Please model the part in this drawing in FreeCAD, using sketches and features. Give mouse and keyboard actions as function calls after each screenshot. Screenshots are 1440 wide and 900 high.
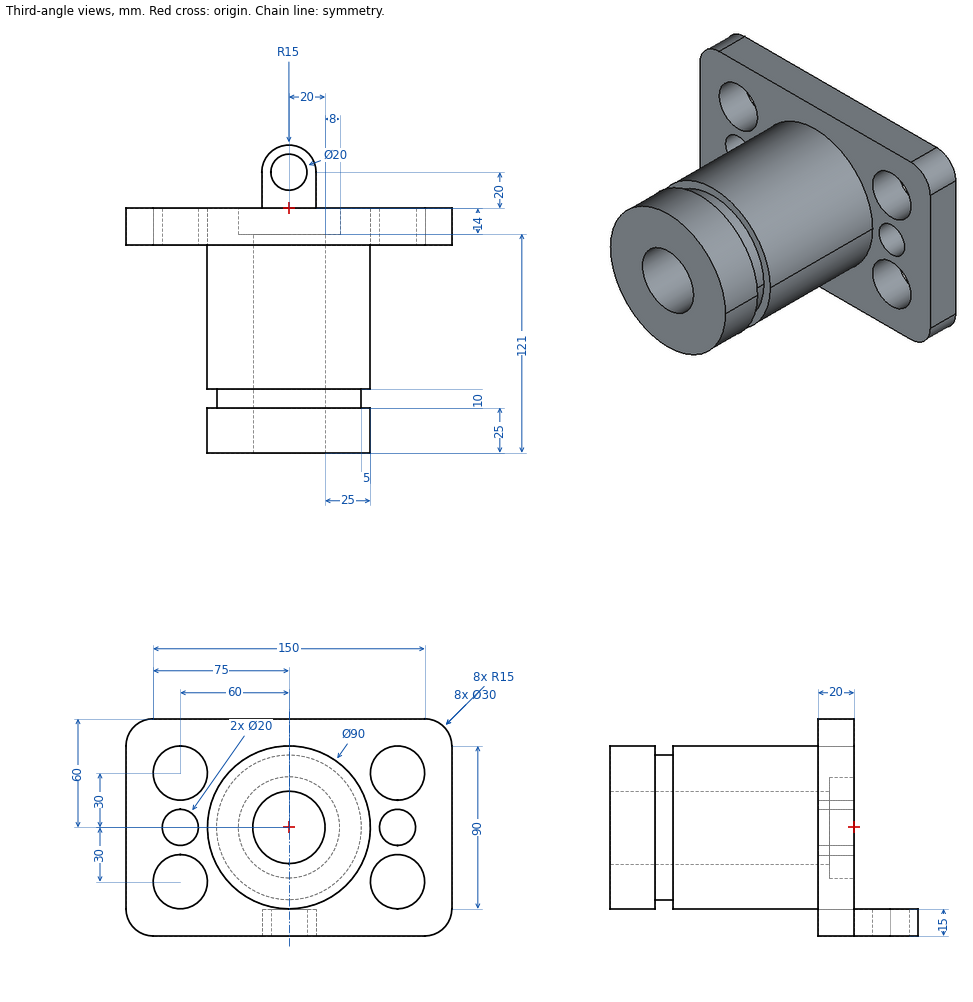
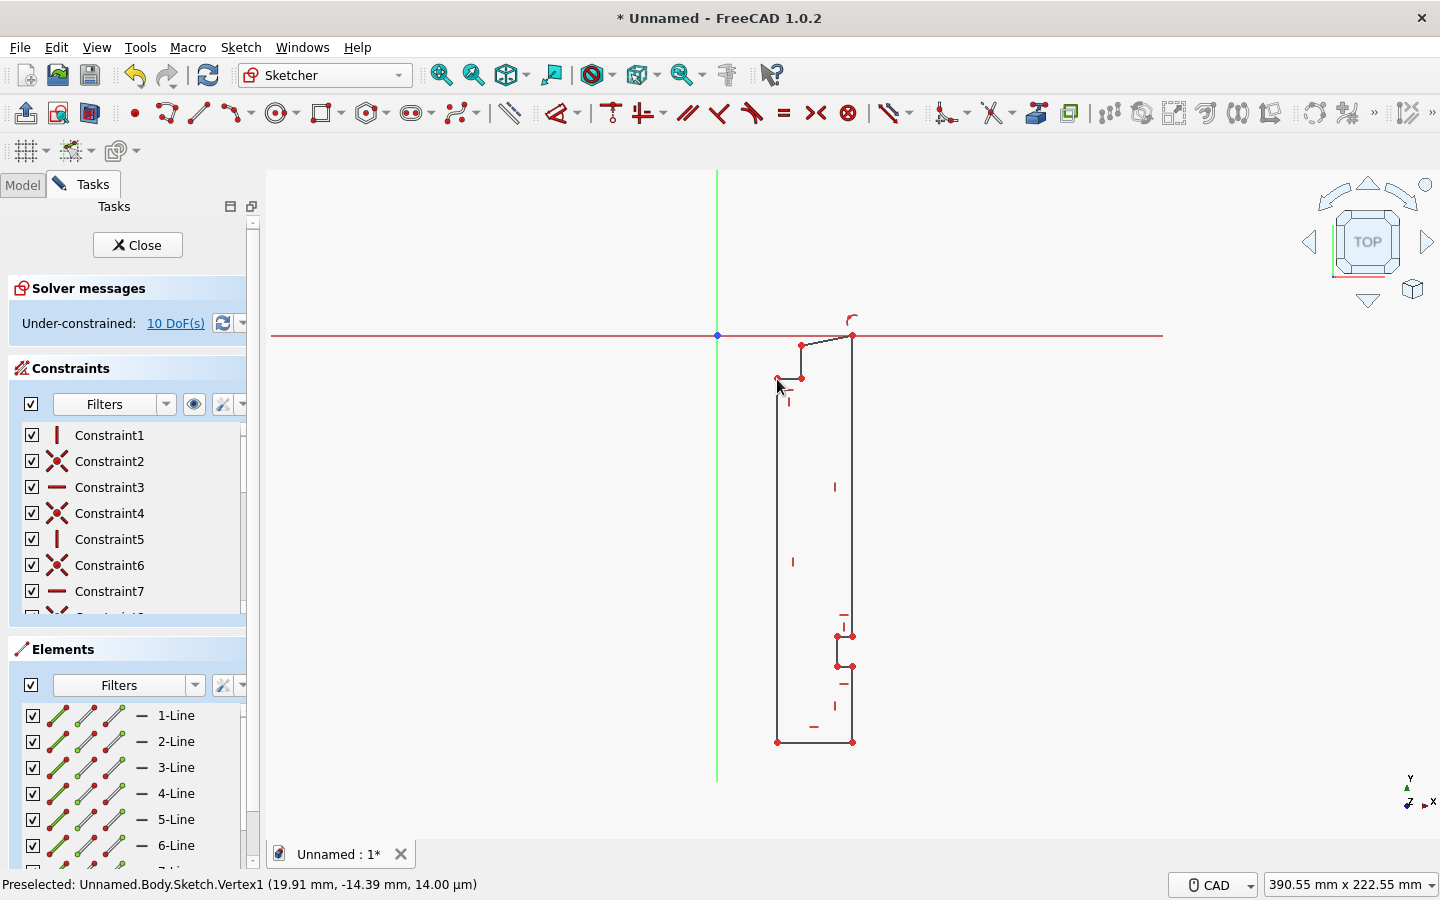
click(837, 339)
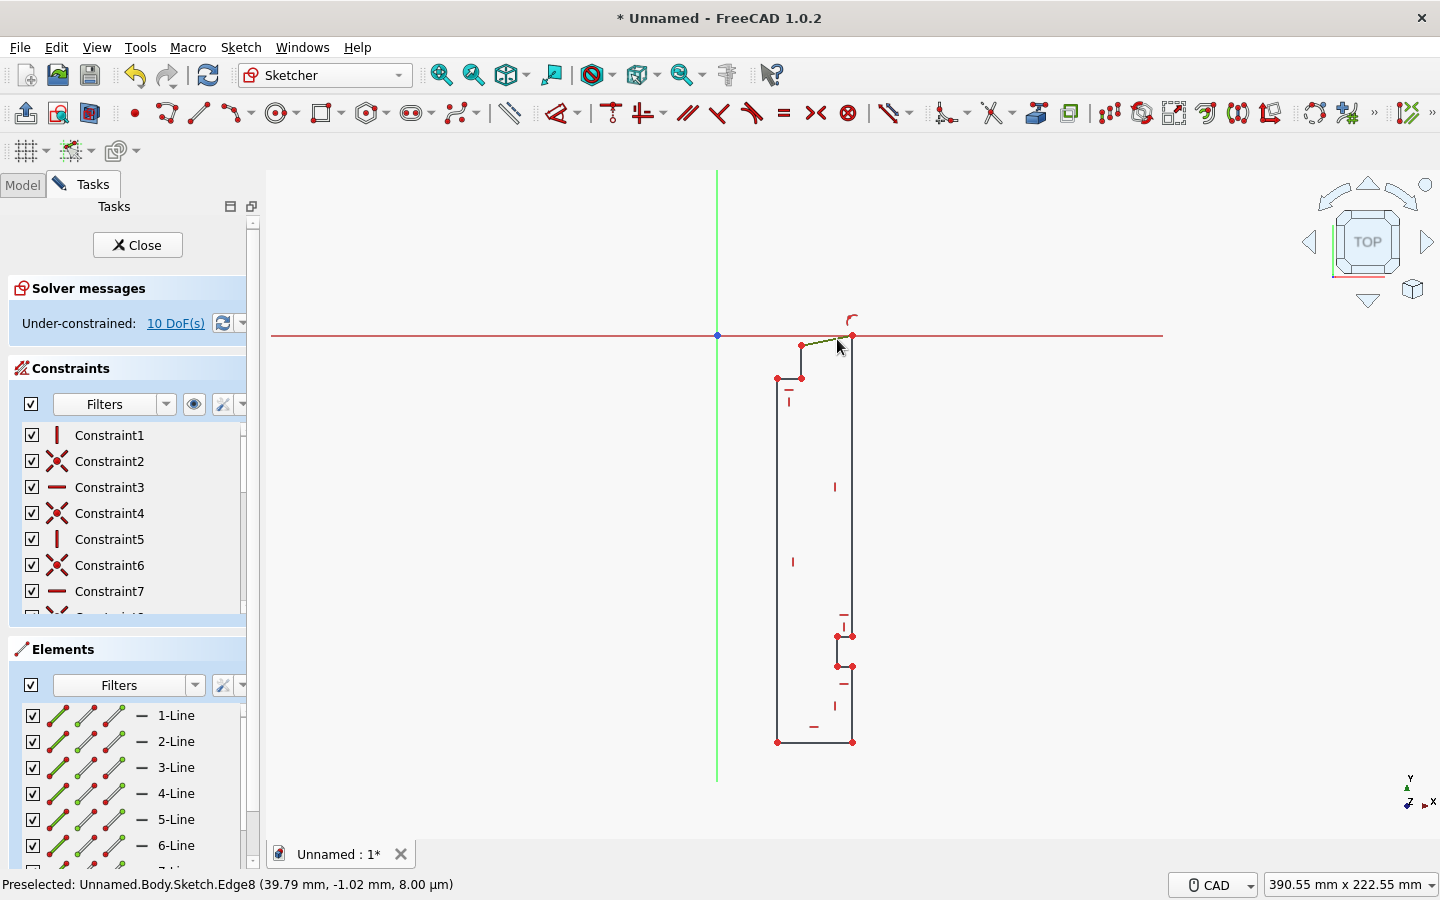
key(h)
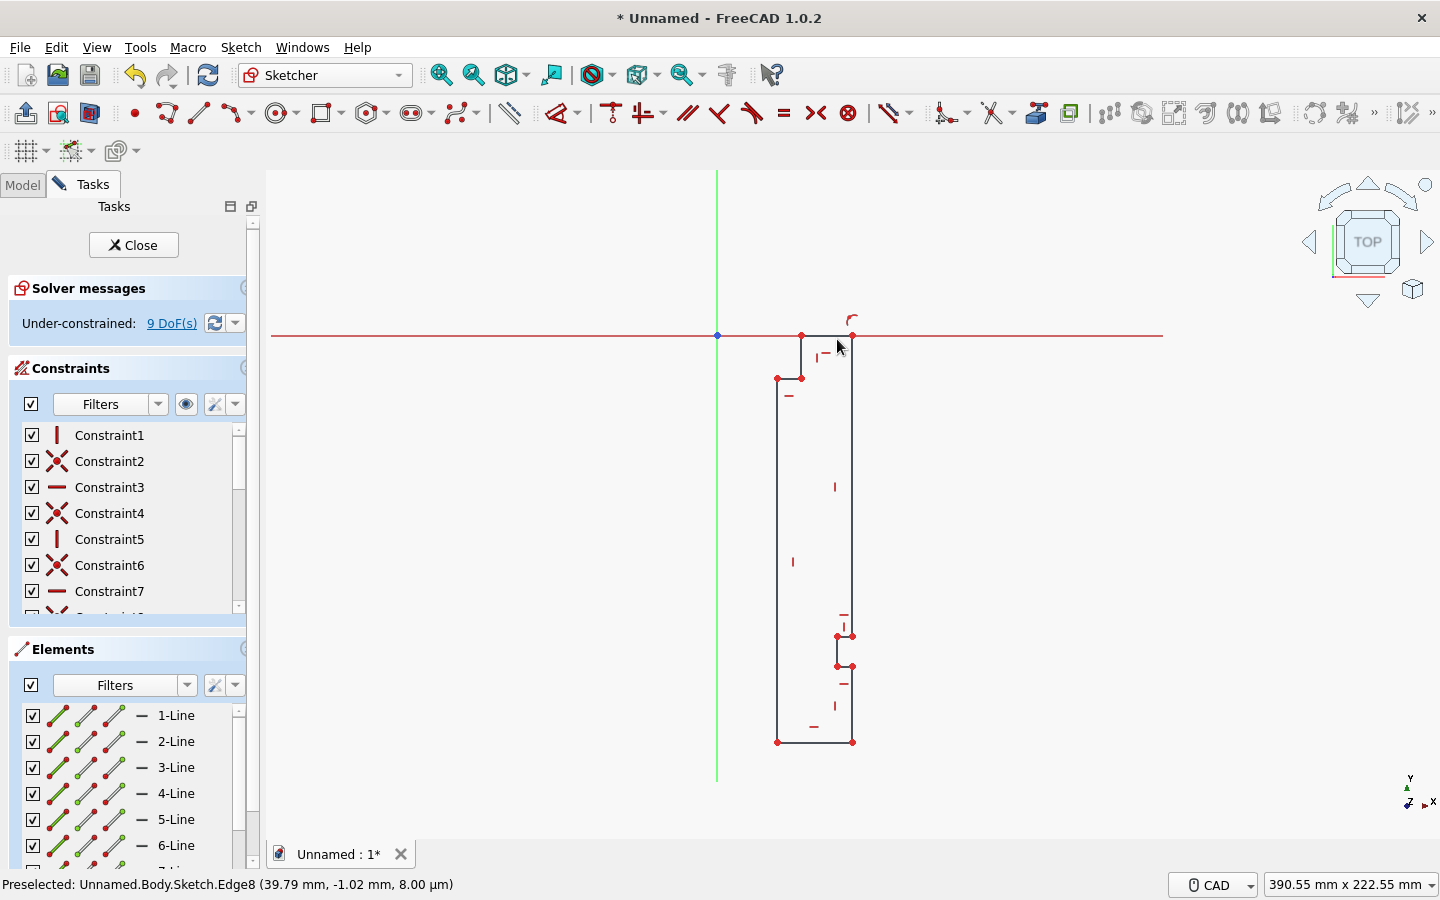
click(556, 114)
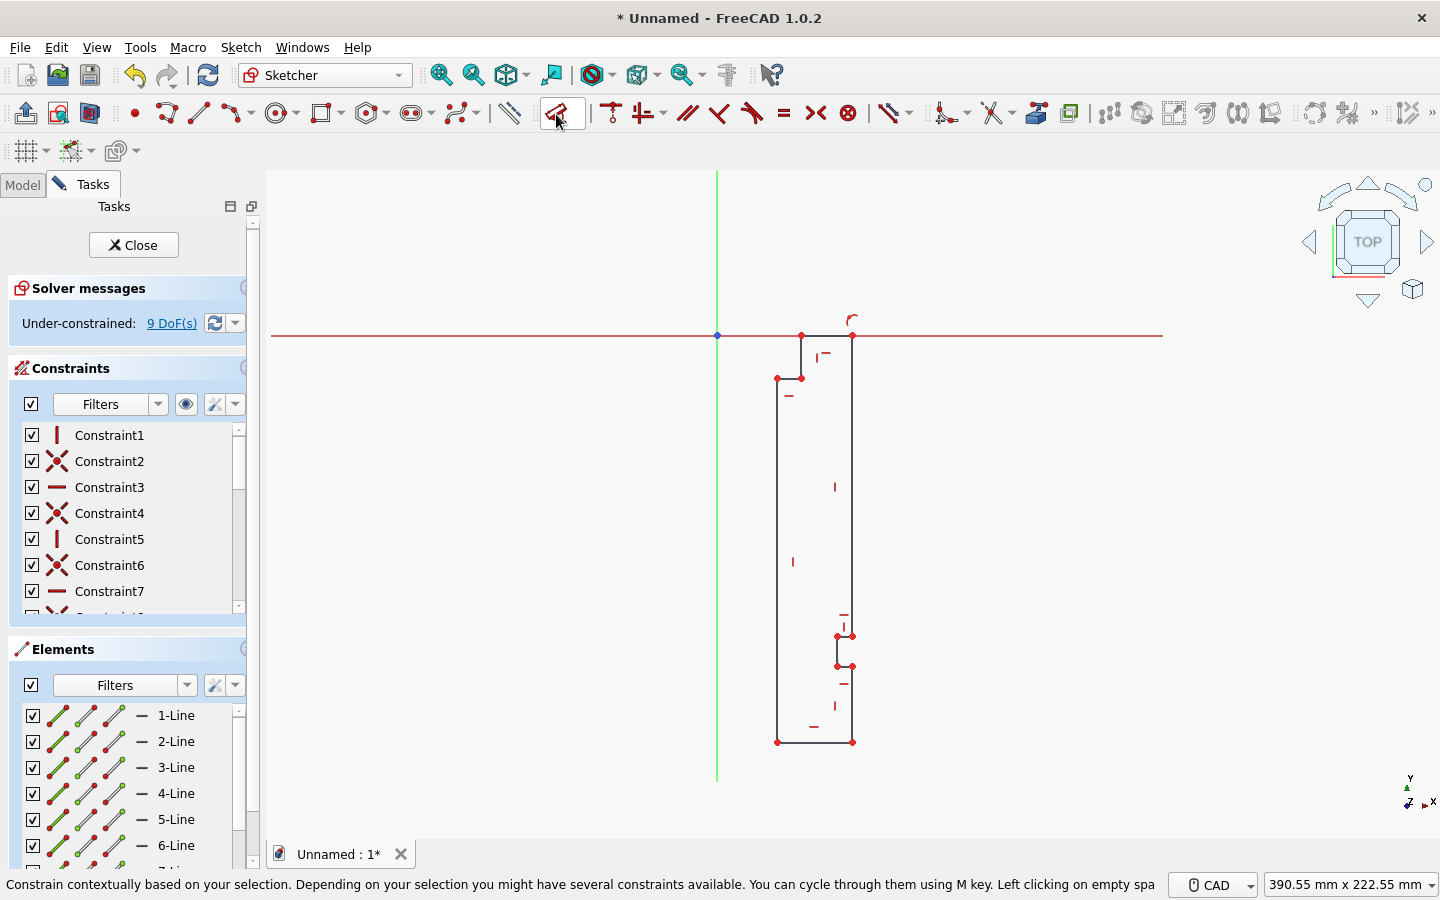
scroll(845, 667, up, 5)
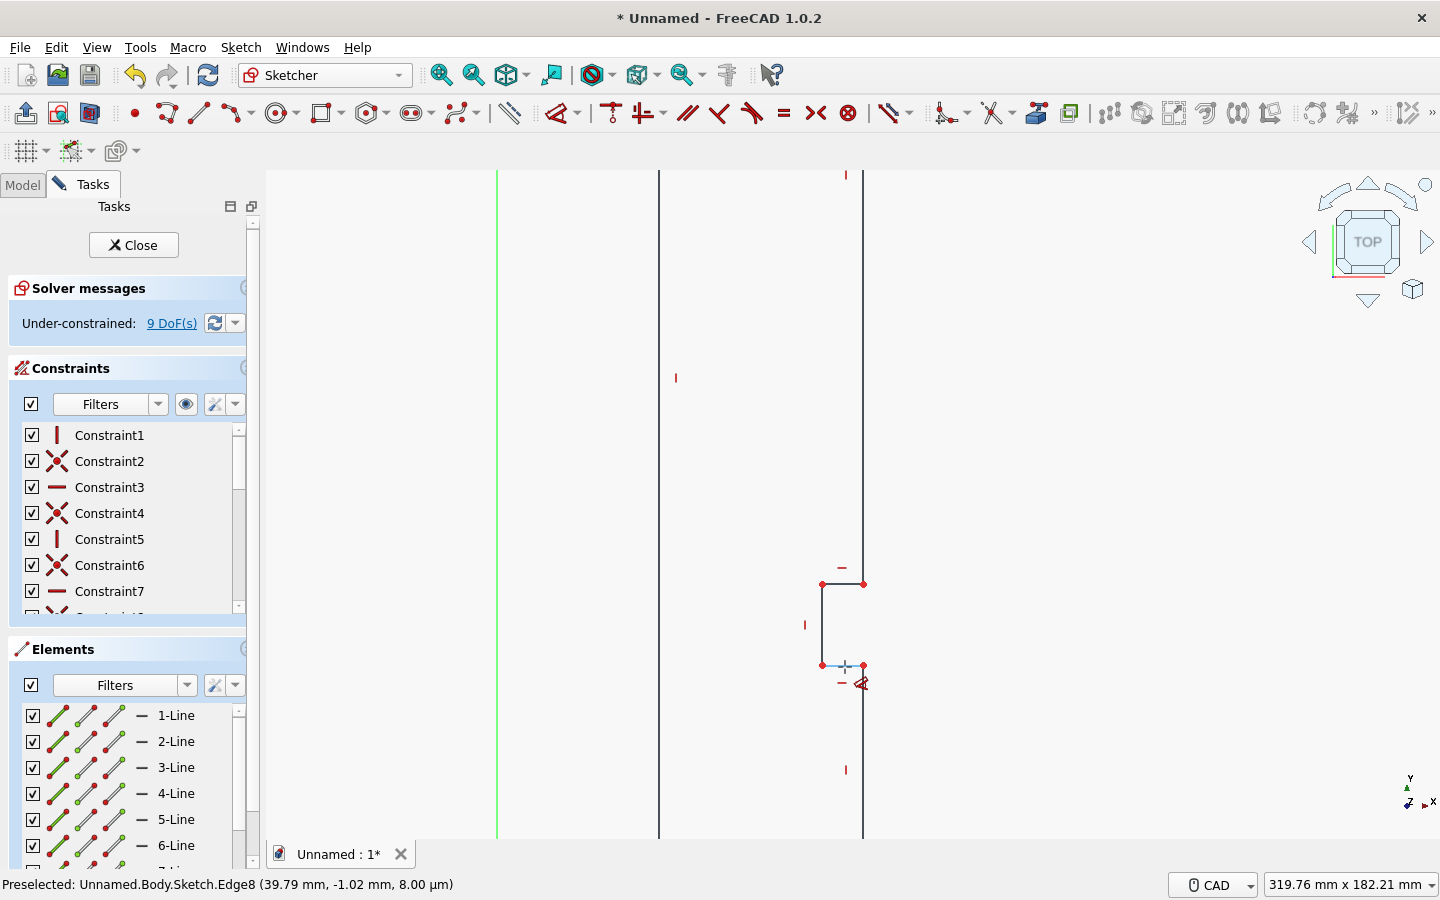
click(843, 666)
click(843, 700)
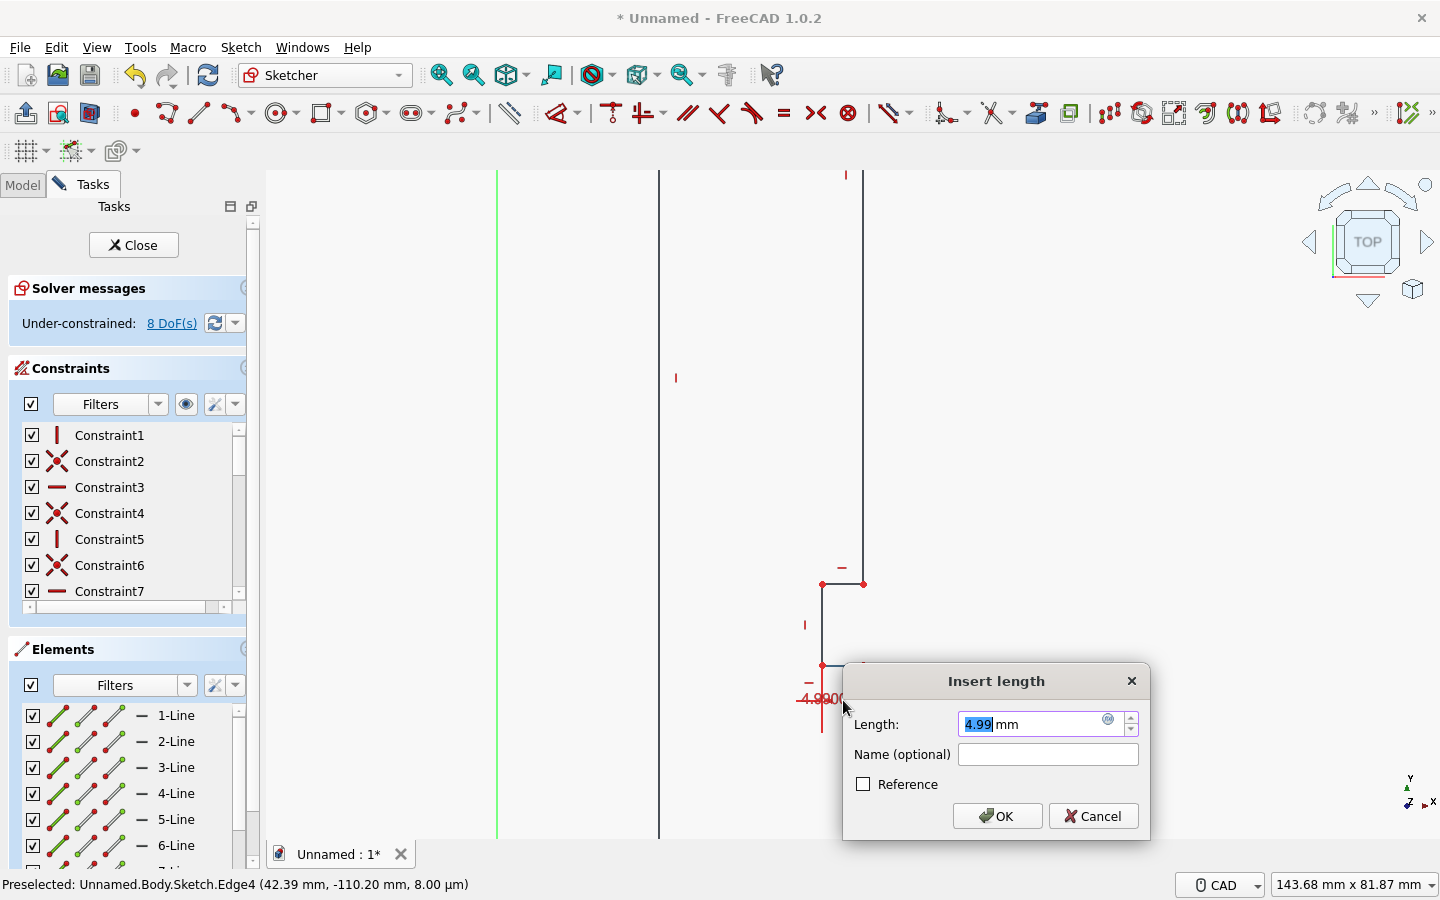
text(5)
key(Return)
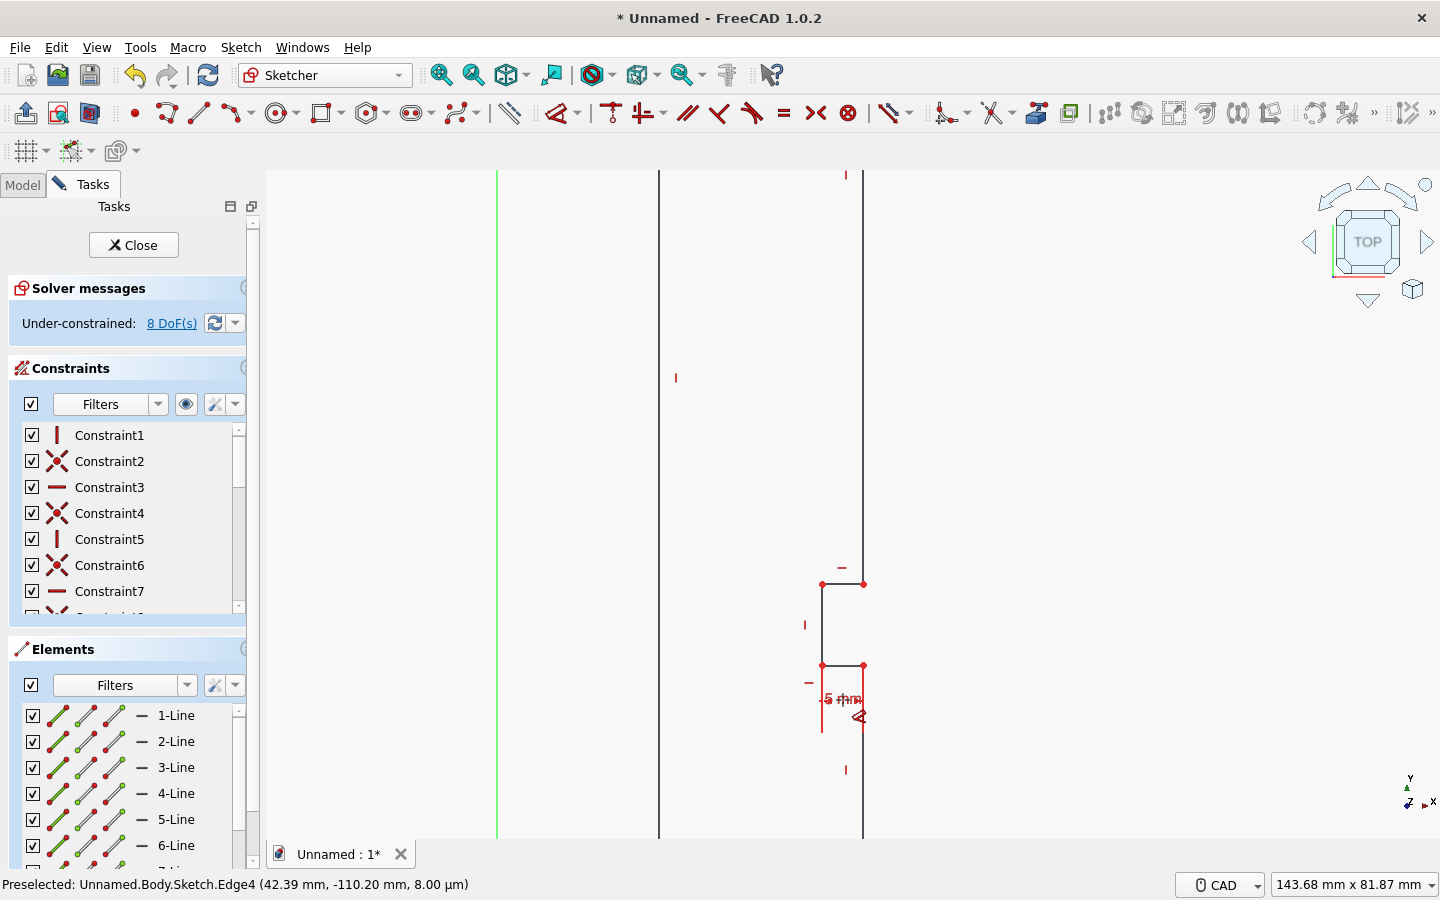
click(835, 584)
click(843, 618)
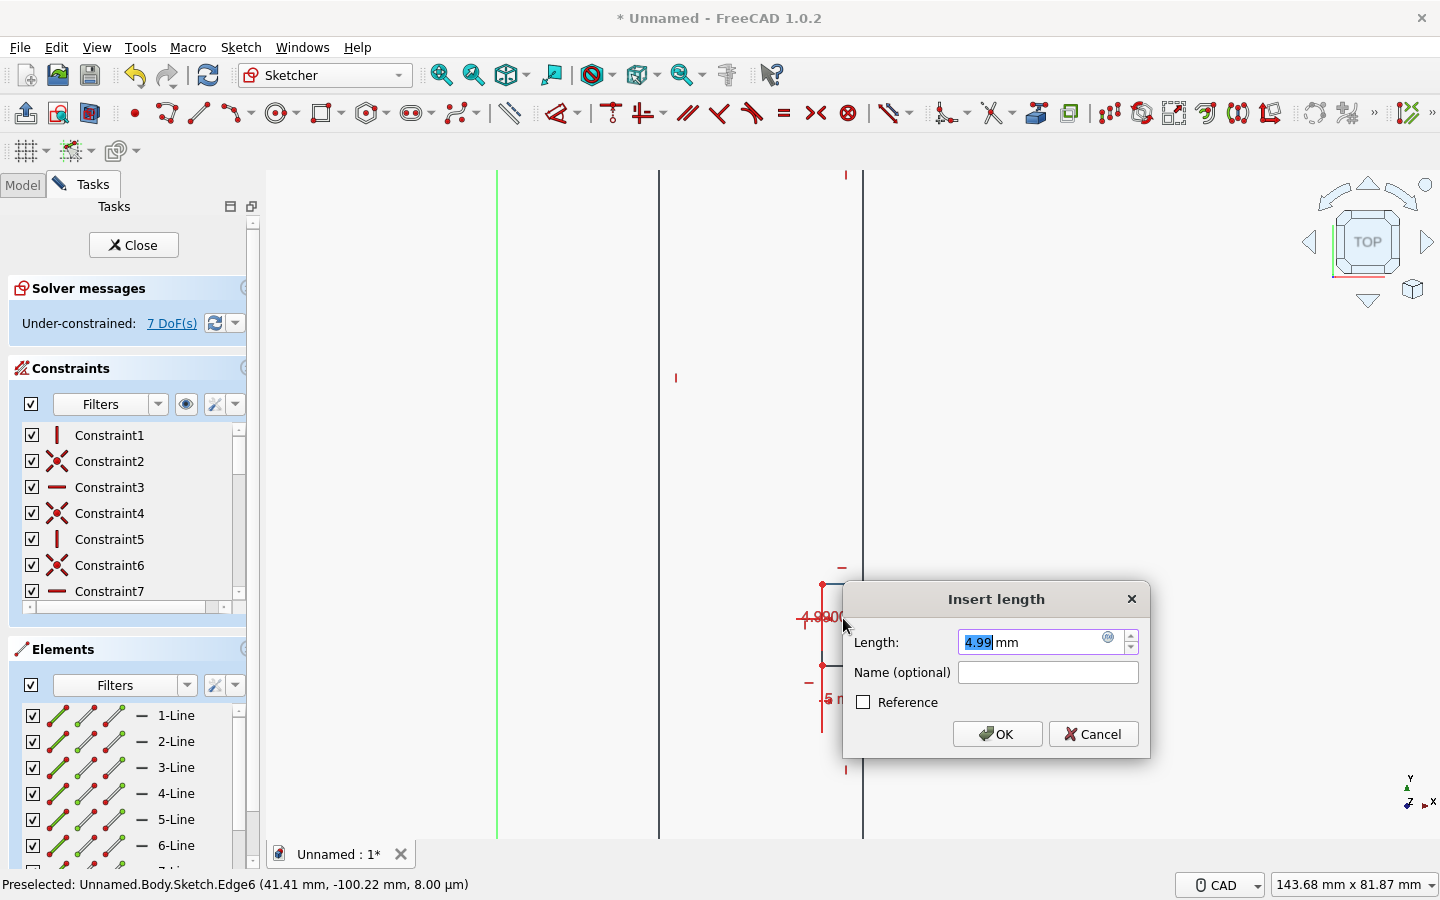
text(5)
key(Return)